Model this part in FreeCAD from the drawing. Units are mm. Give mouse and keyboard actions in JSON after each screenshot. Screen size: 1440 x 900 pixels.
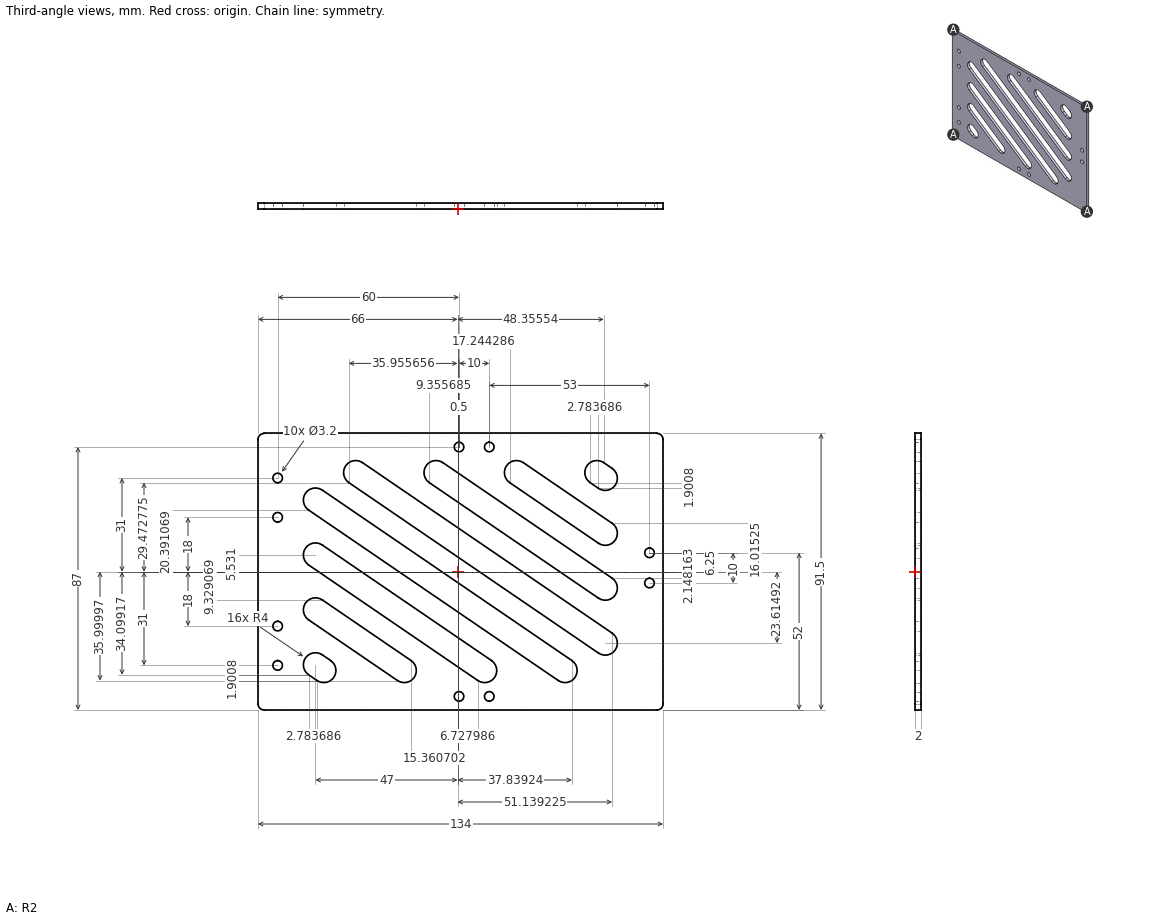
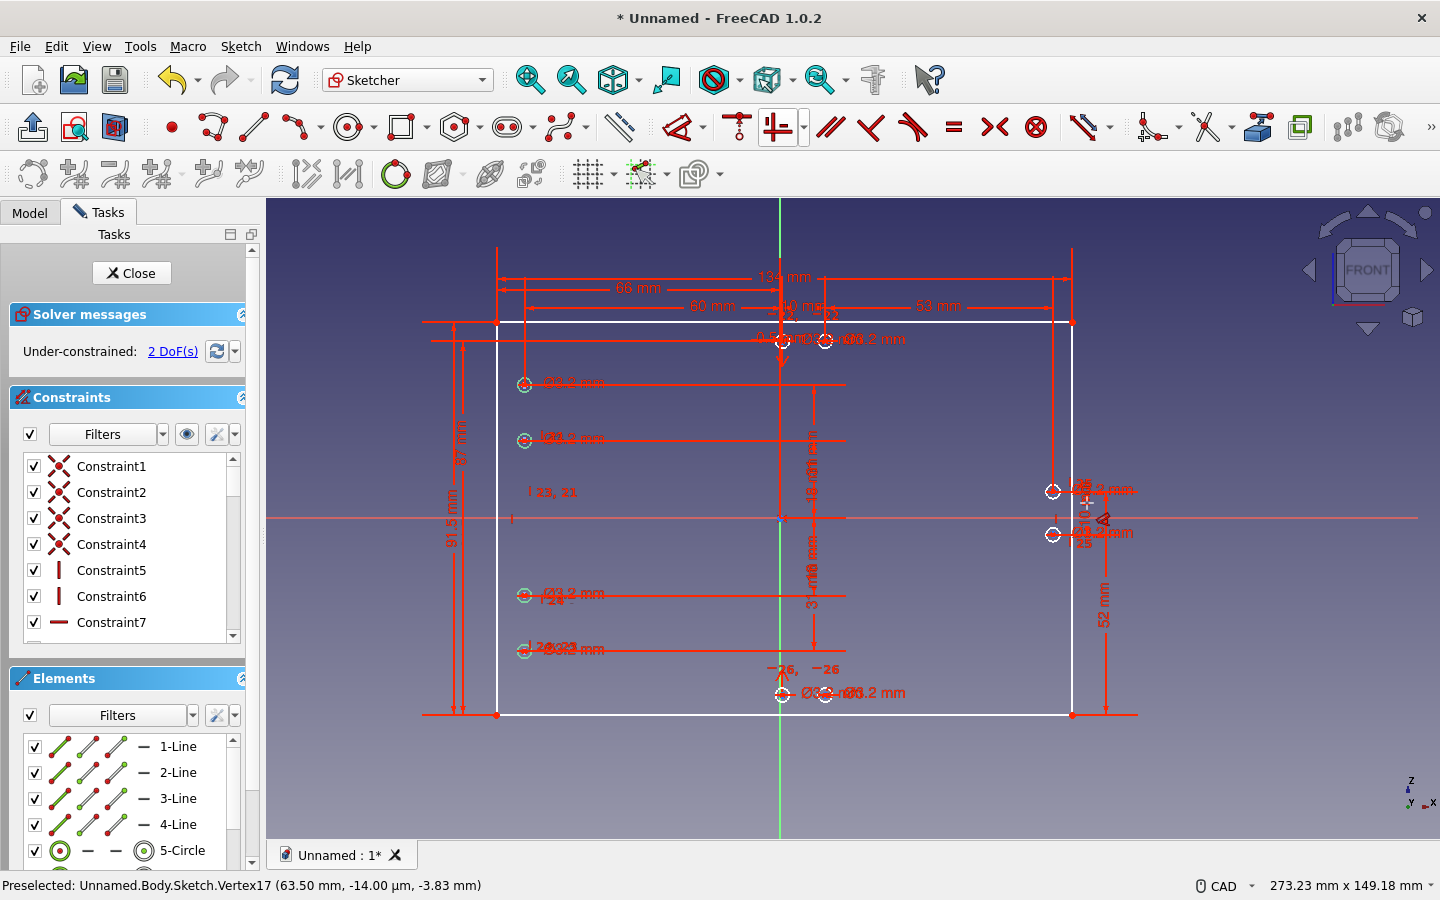
{"action": "left_click", "coordinate": [782, 695]}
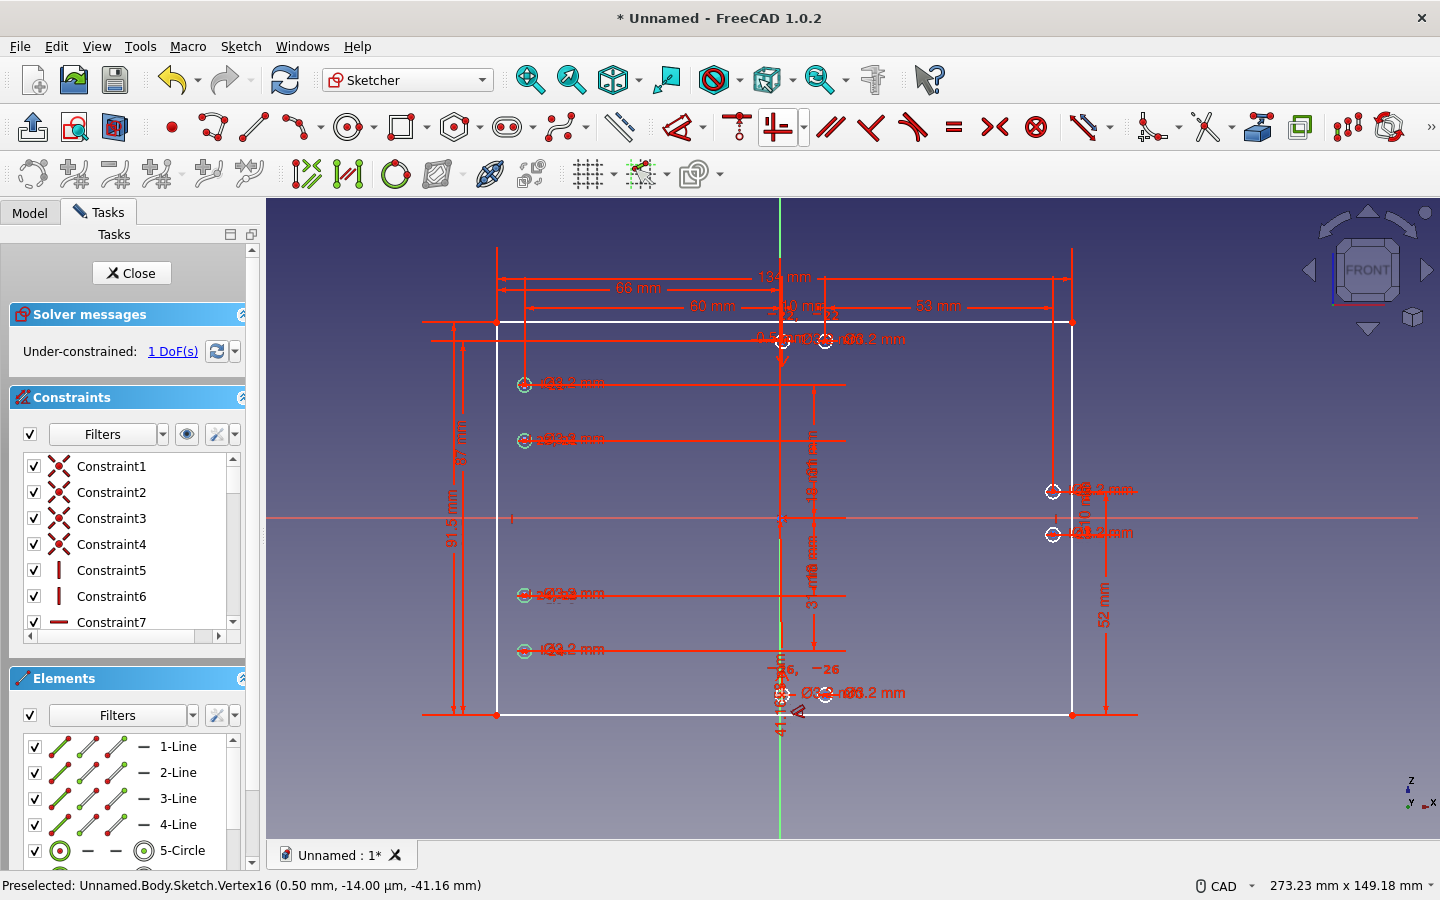
{"action": "left_click", "coordinate": [825, 695]}
{"action": "left_click", "coordinate": [804, 729]}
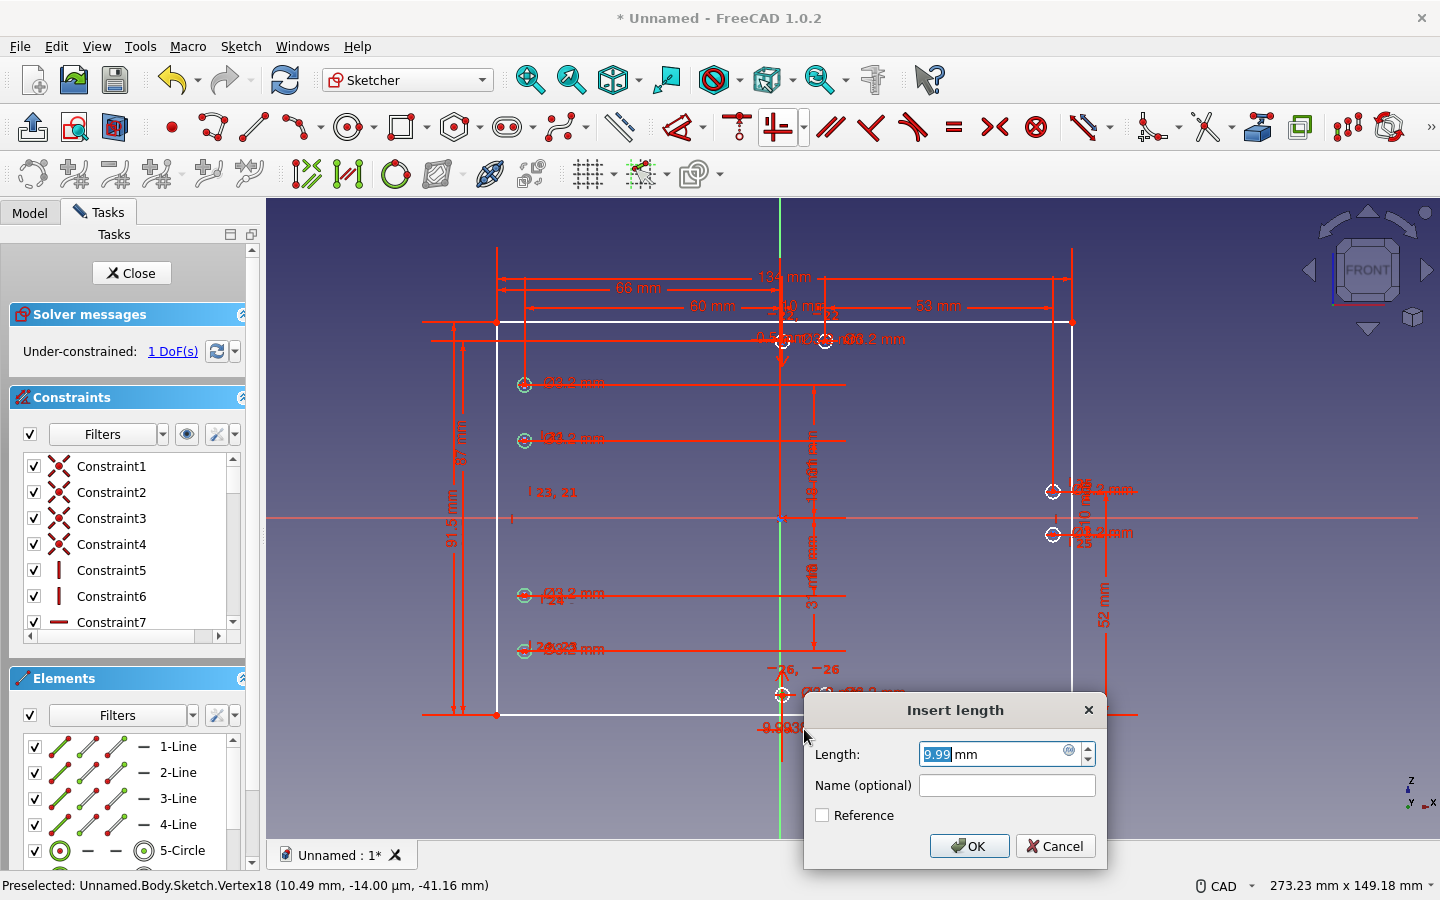
{"action": "type", "text": "10"}
{"action": "key", "text": "Return"}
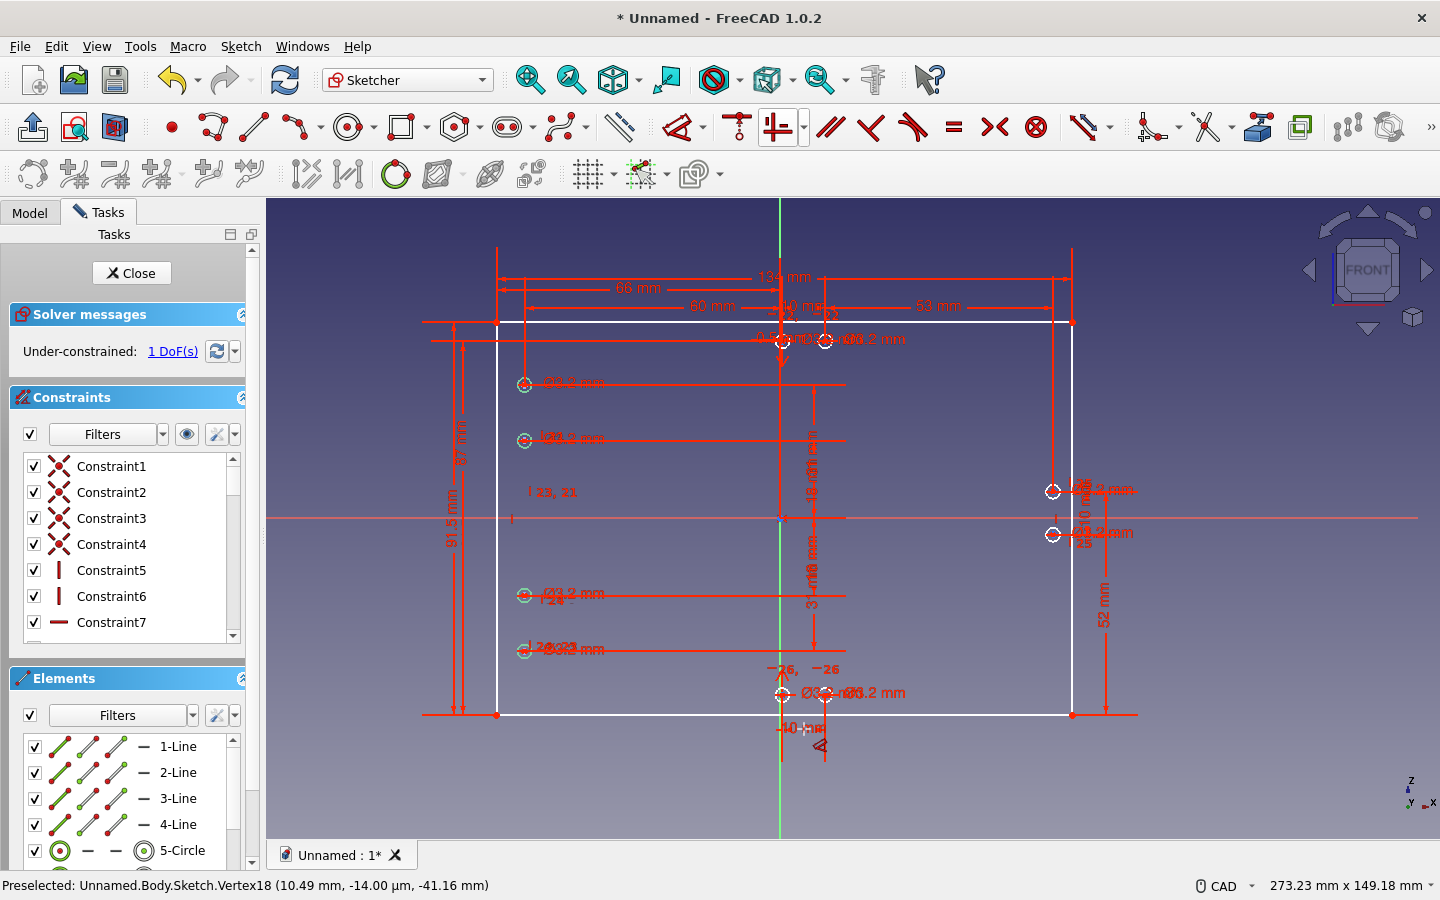
{"action": "scroll", "coordinate": [1053, 492], "scroll_direction": "up", "scroll_amount": 2}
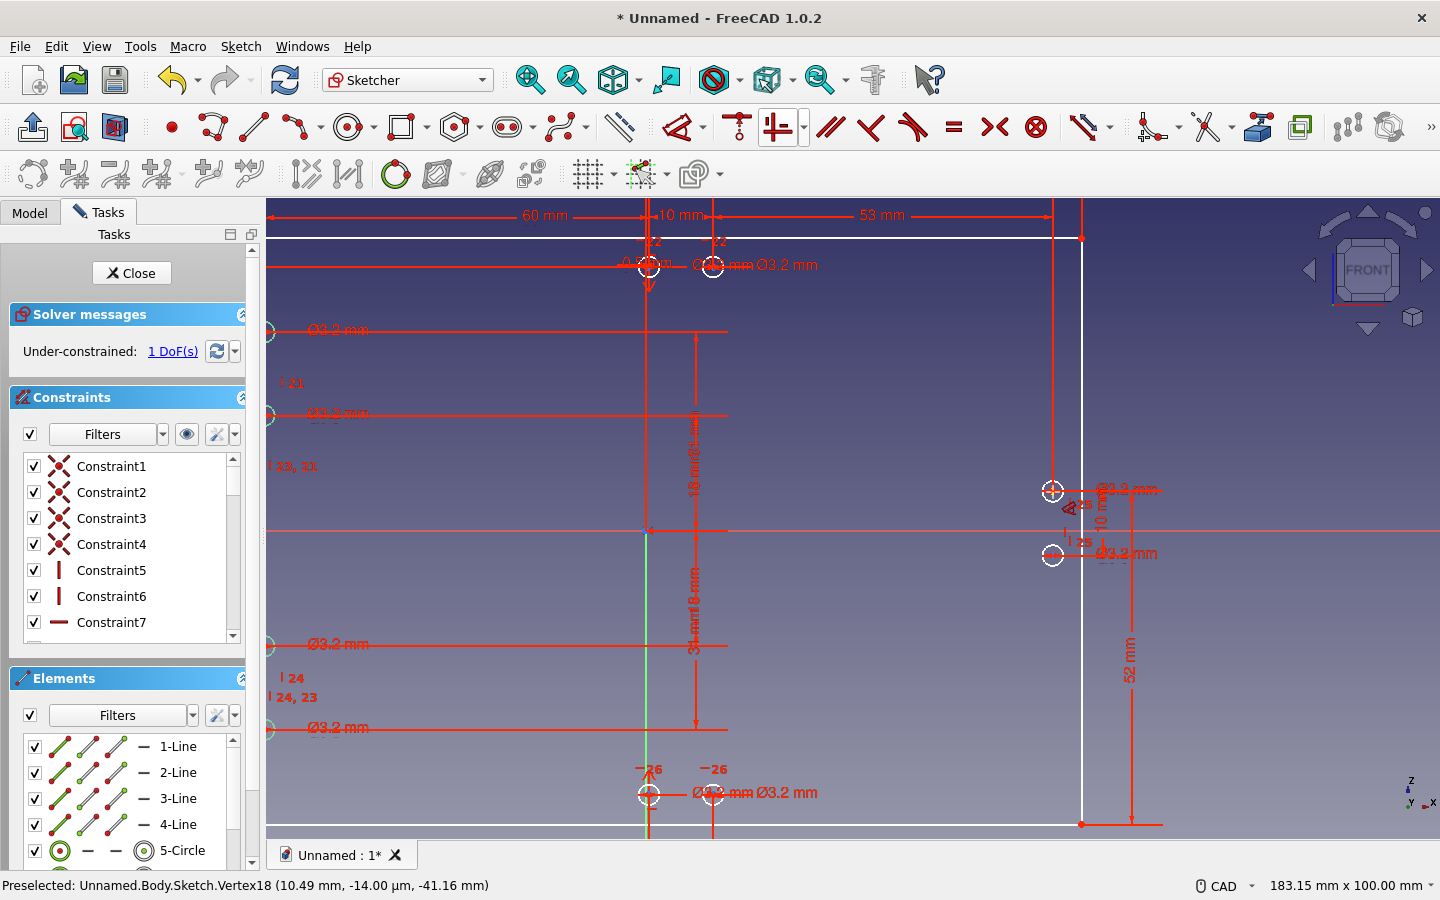
{"action": "left_click", "coordinate": [1053, 491]}
{"action": "left_click", "coordinate": [612, 511]}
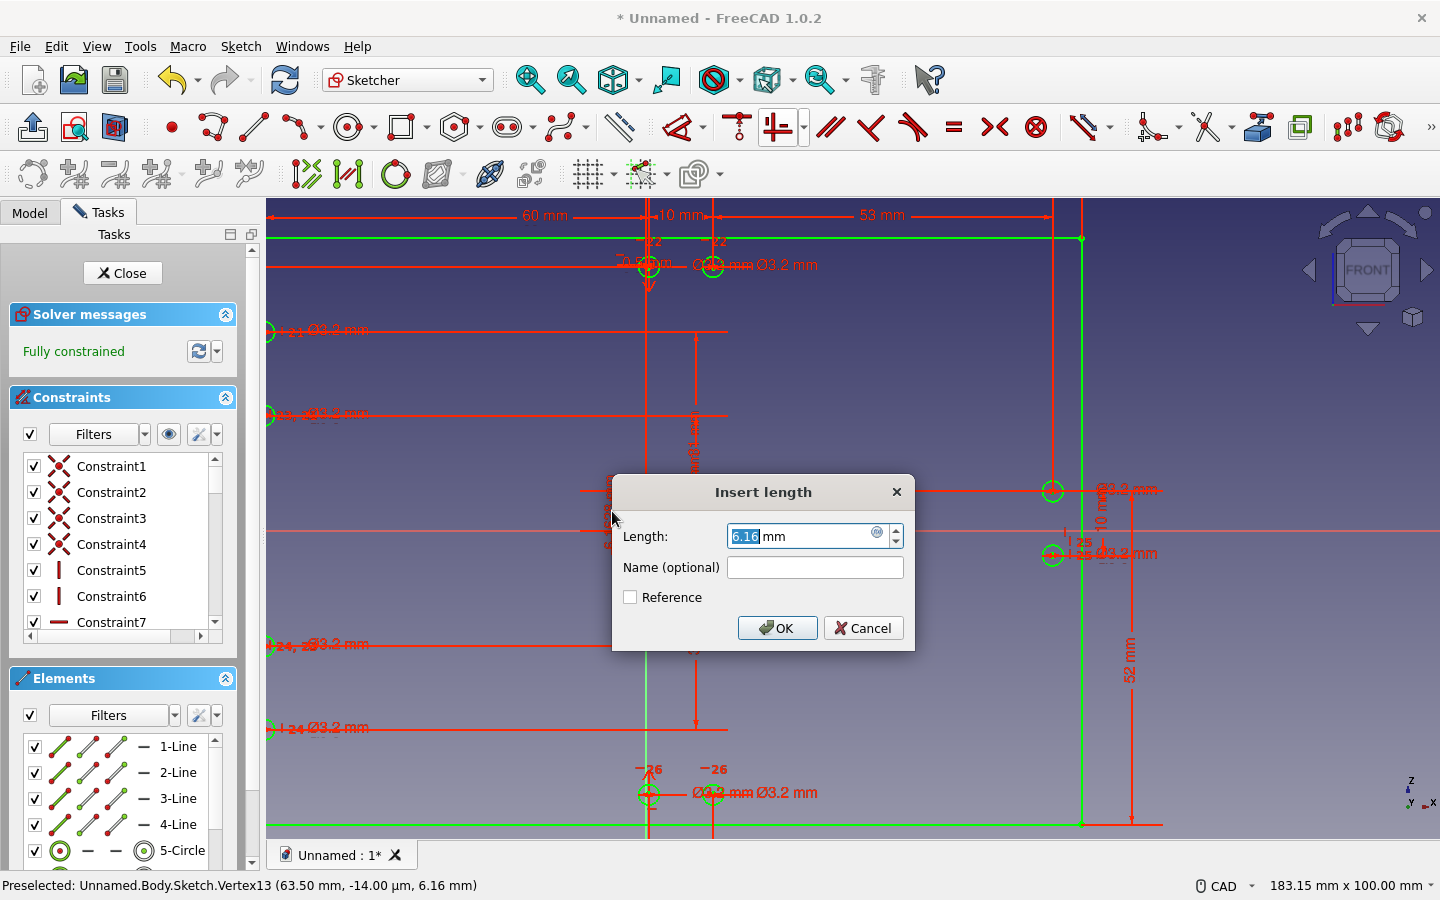
{"action": "type", "text": "6.25"}
{"action": "key", "text": "Return"}
{"action": "key", "text": "Escape"}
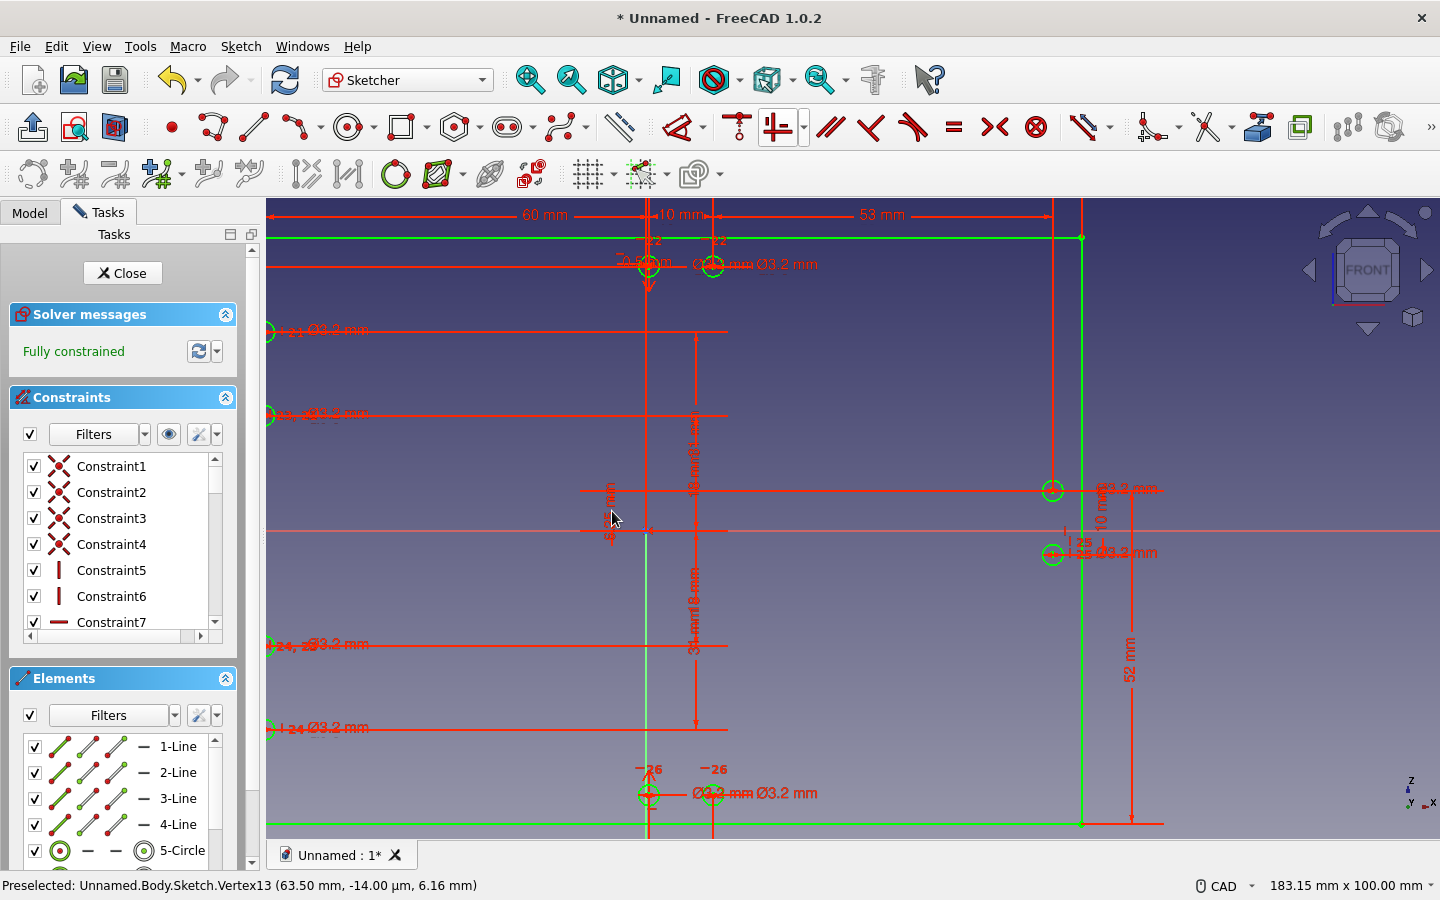
{"action": "left_click", "coordinate": [123, 273]}